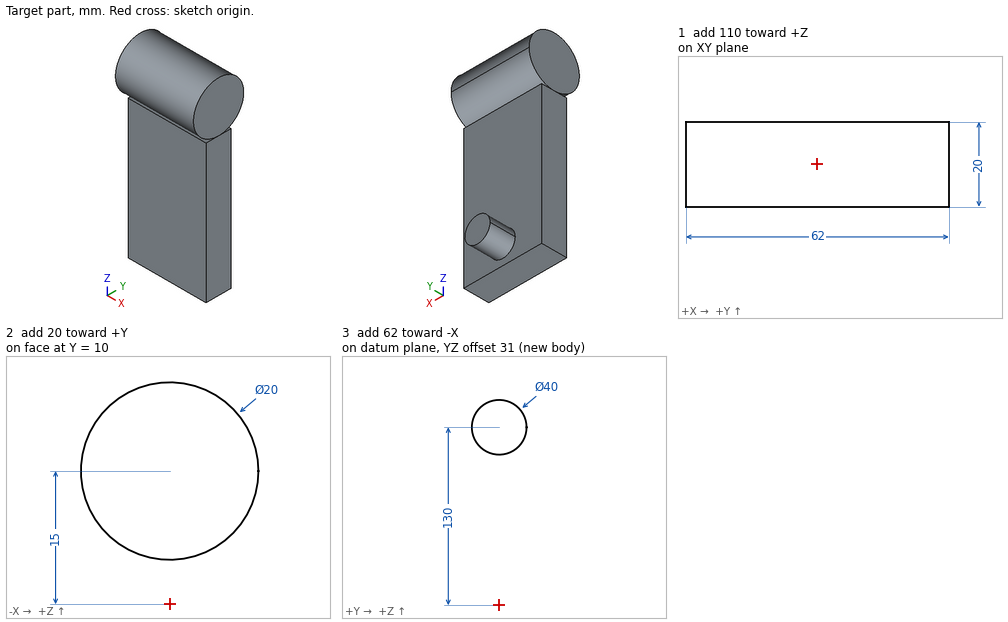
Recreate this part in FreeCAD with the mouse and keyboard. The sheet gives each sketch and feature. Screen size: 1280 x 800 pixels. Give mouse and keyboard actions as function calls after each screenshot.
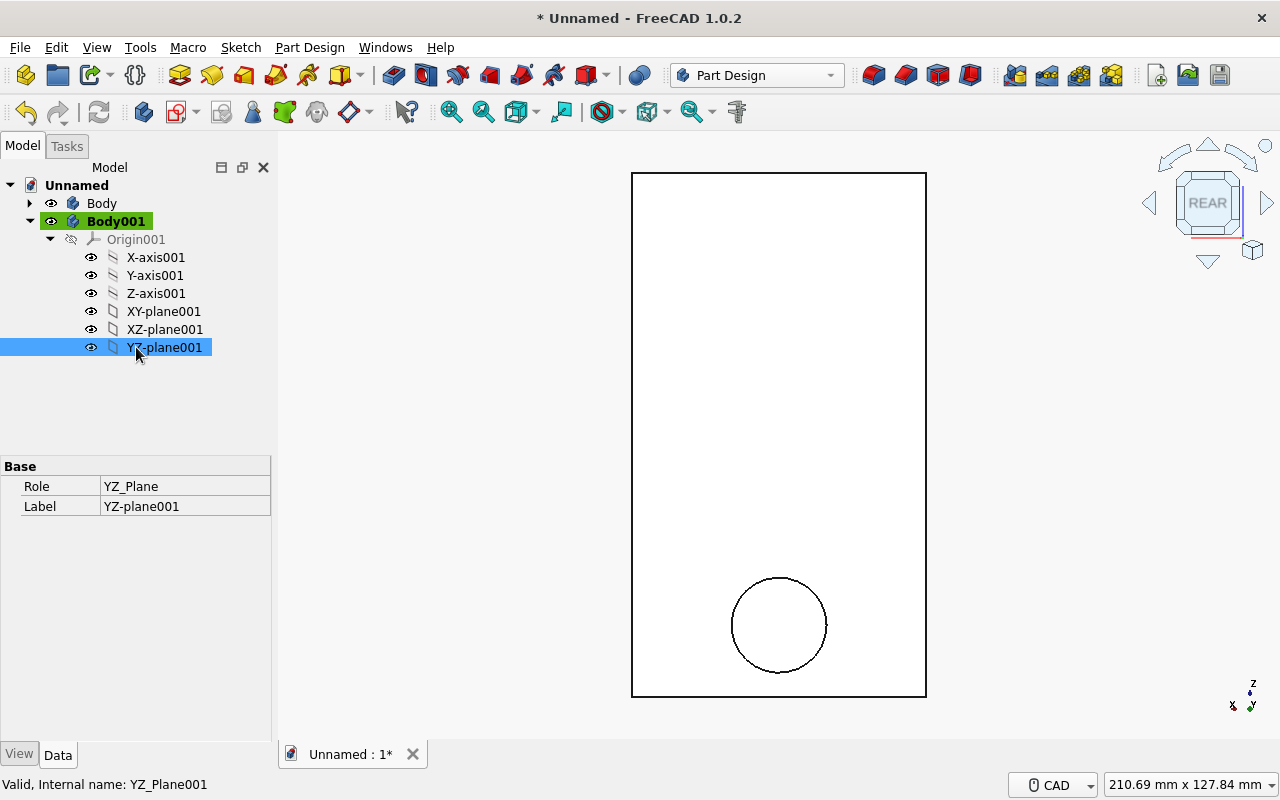
click(350, 112)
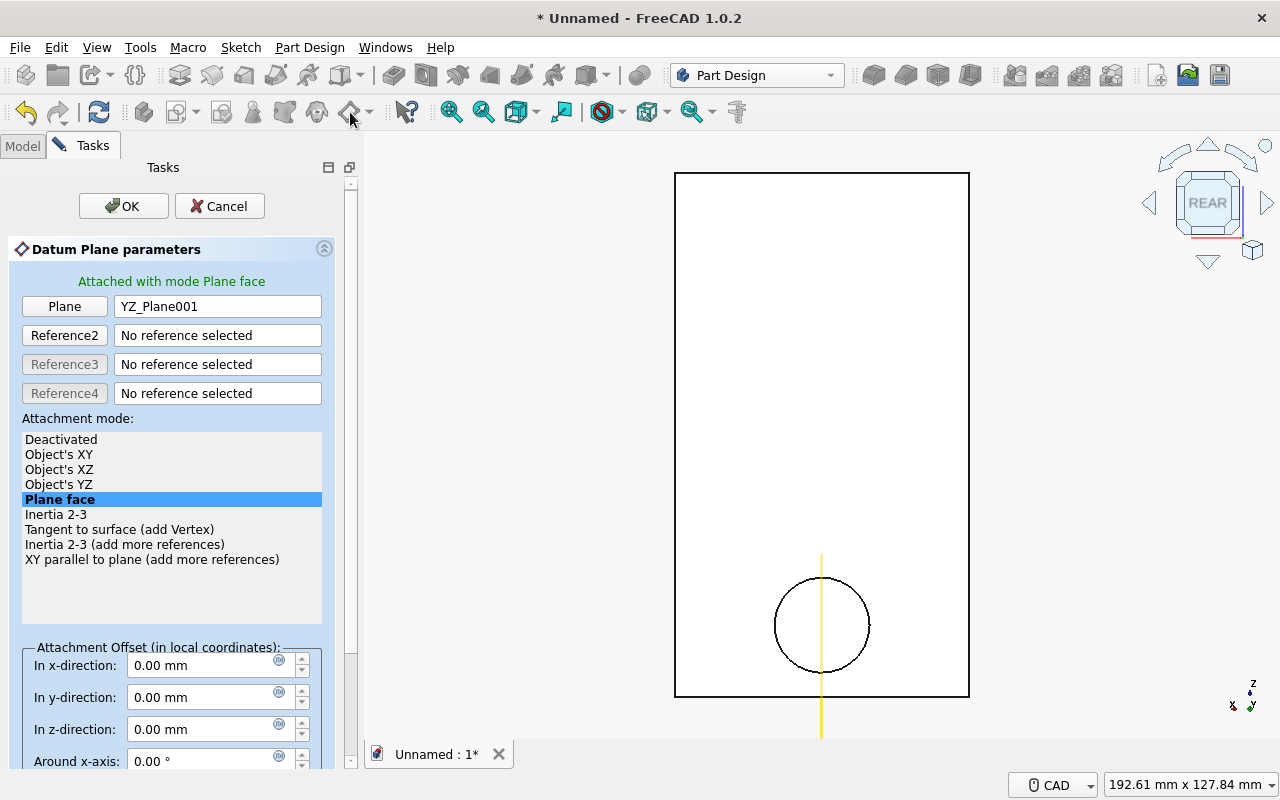
triple_click(210, 729)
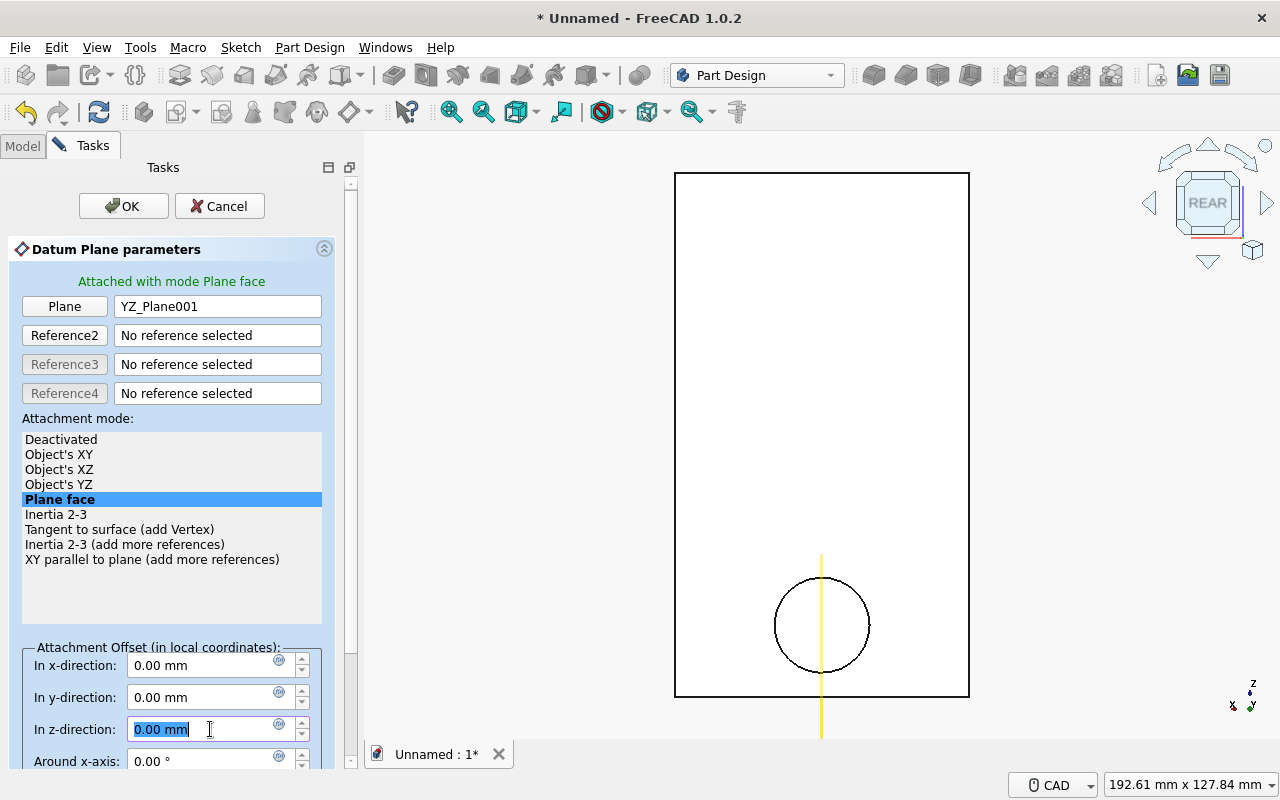
text(31)
key(Tab)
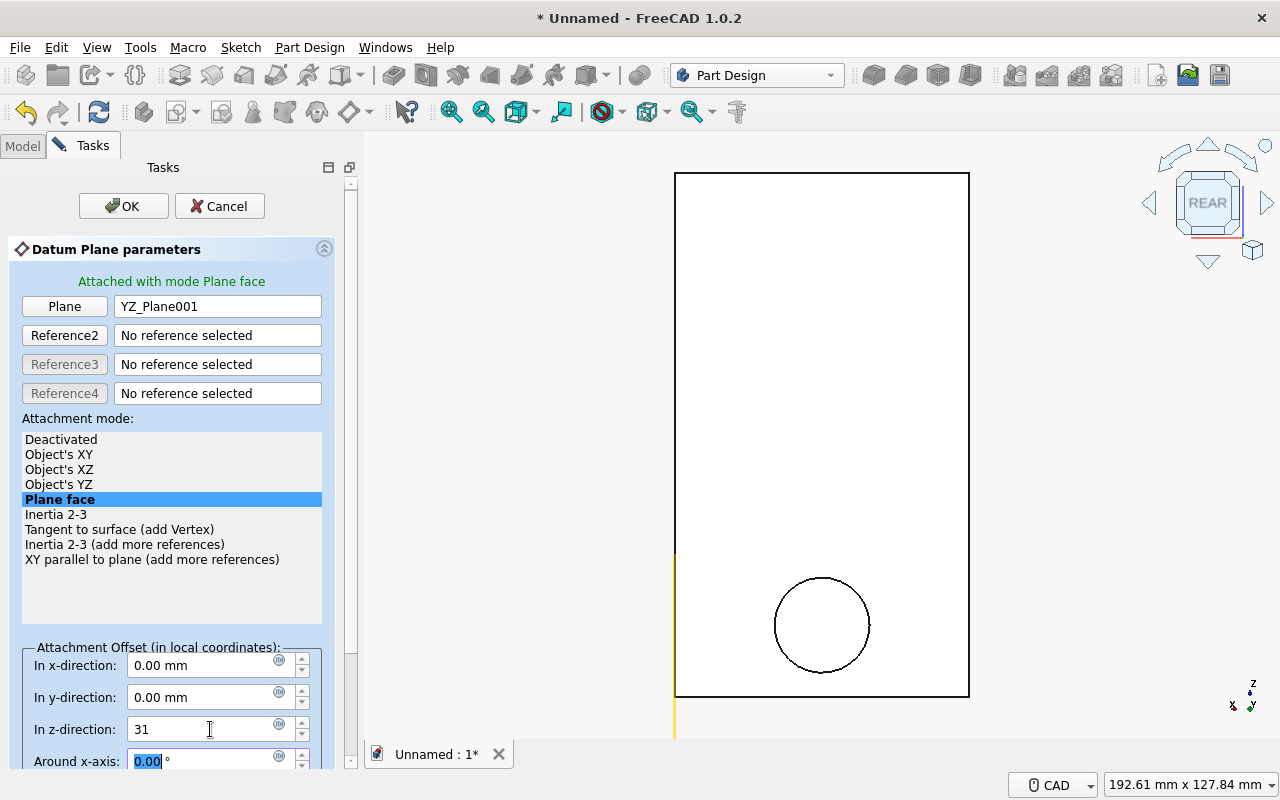
click(124, 206)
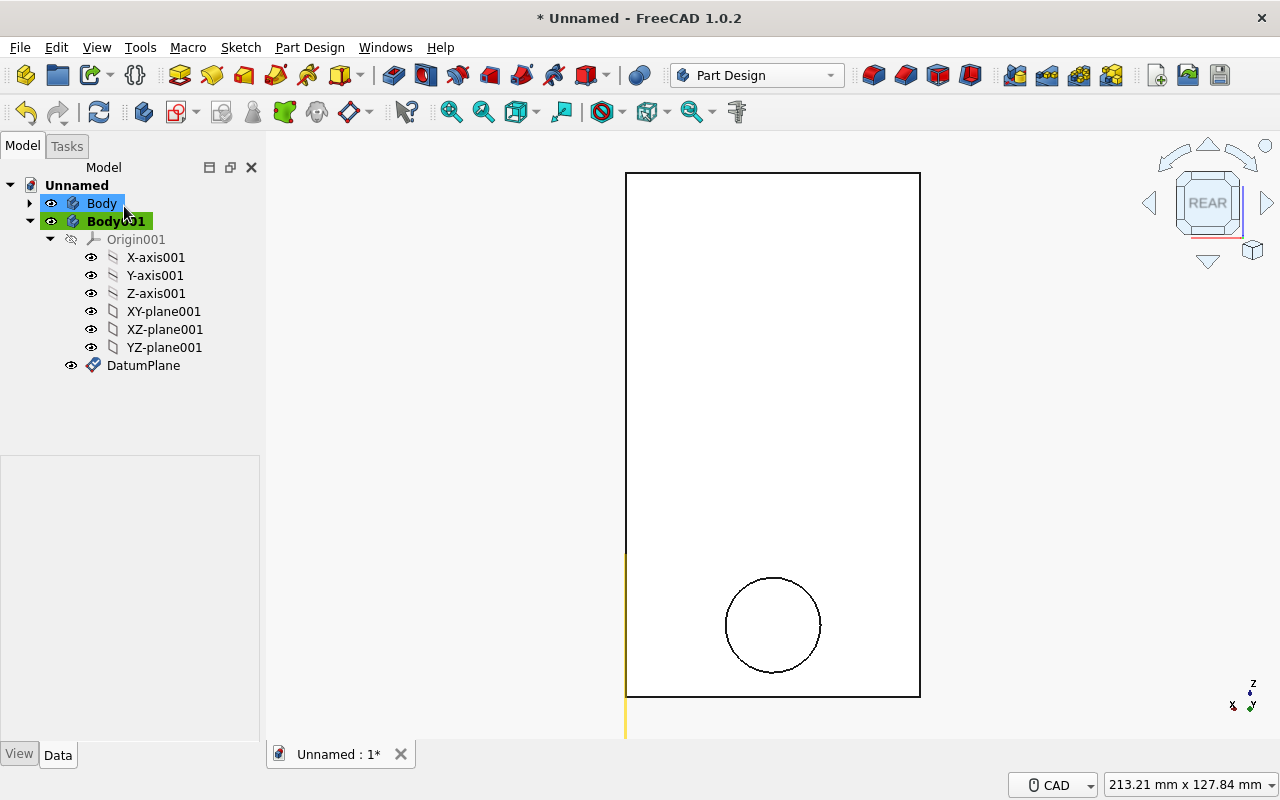
click(116, 365)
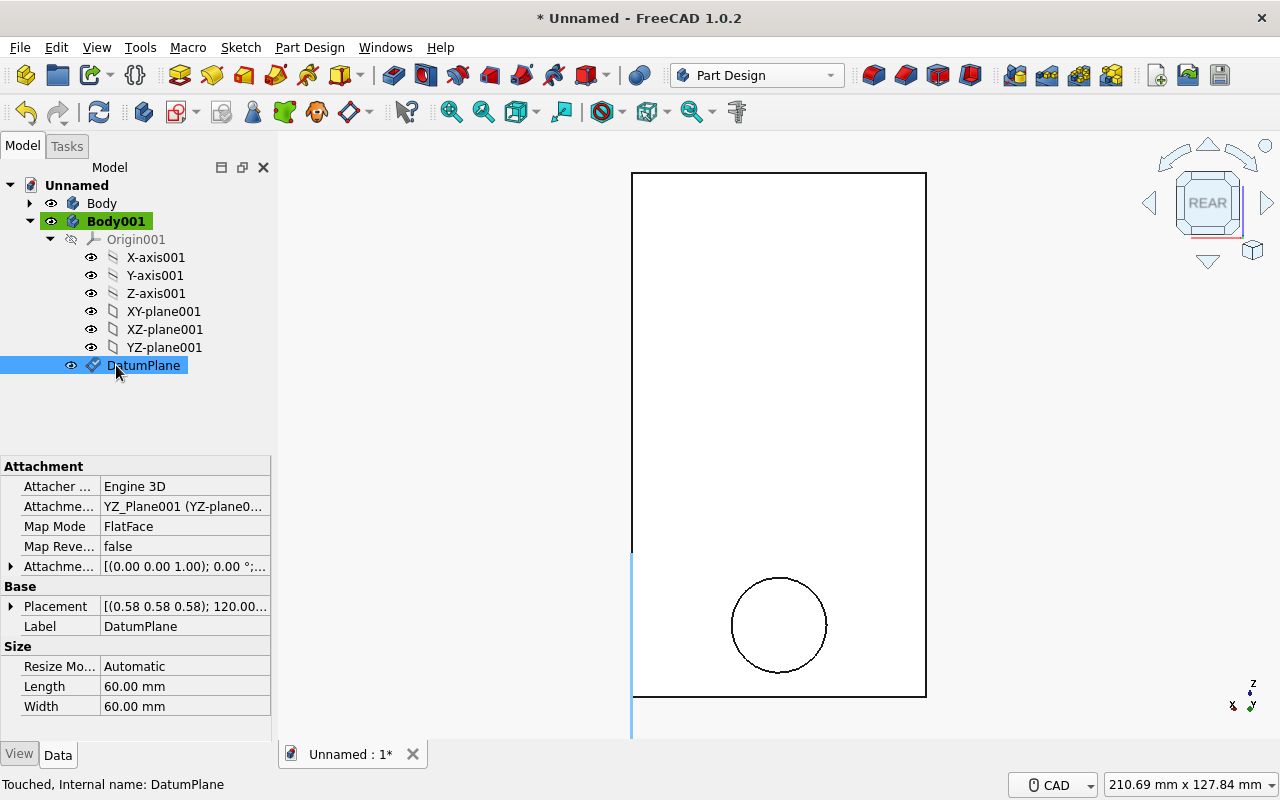
click(176, 112)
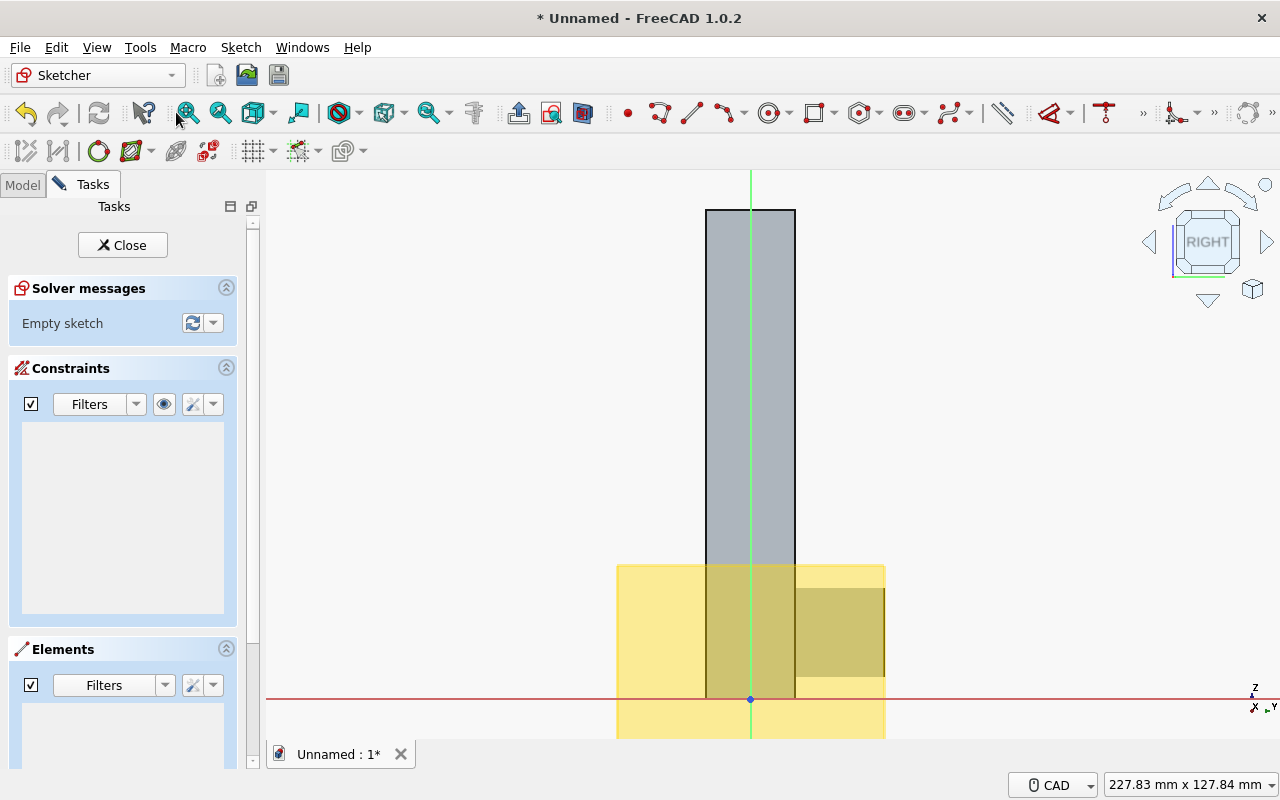
scroll(704, 454, down, 5)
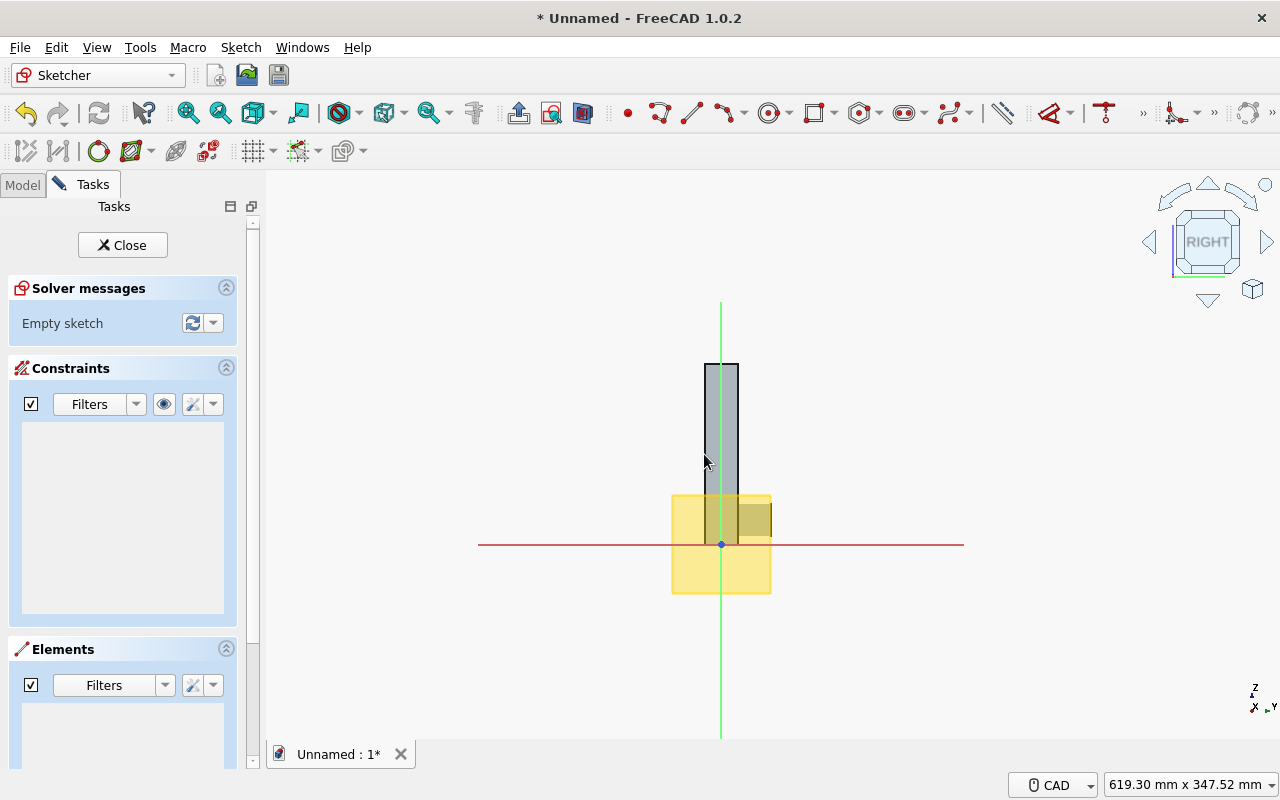
scroll(725, 307, up, 9)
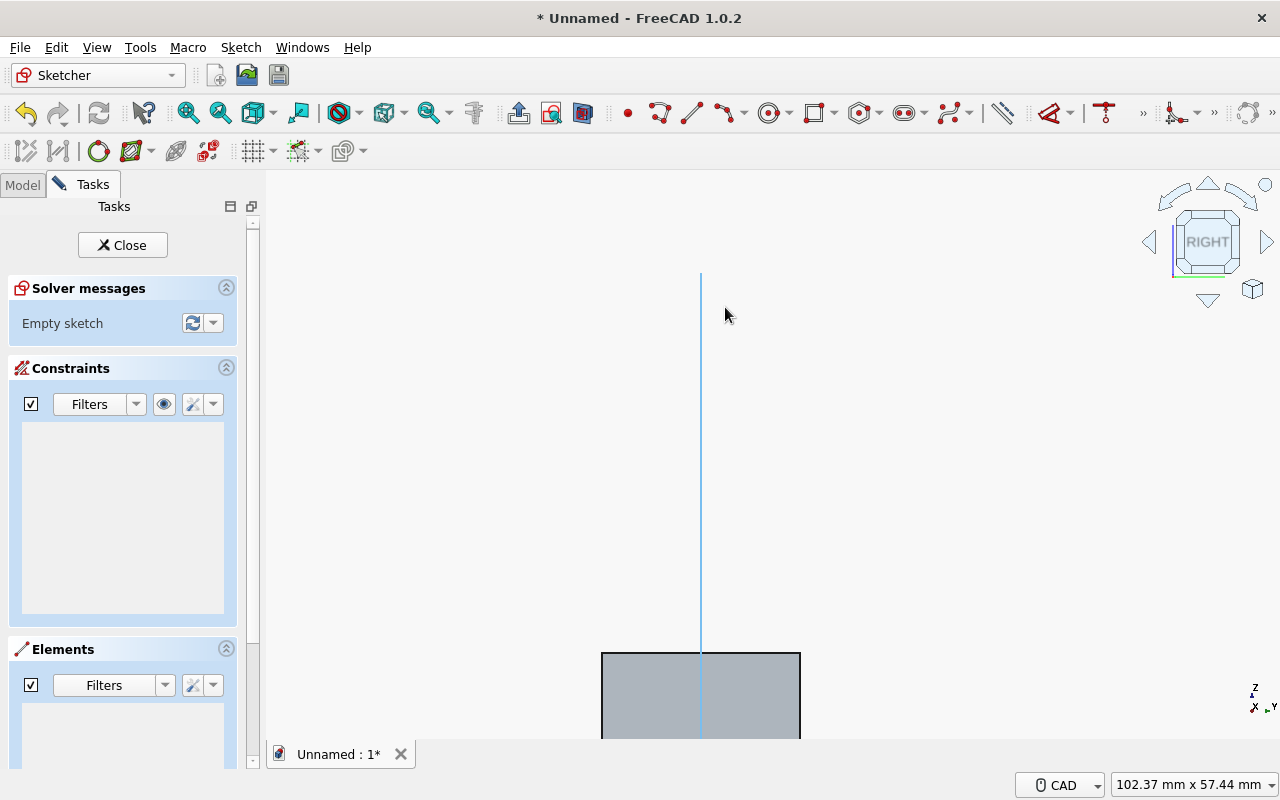
click(770, 114)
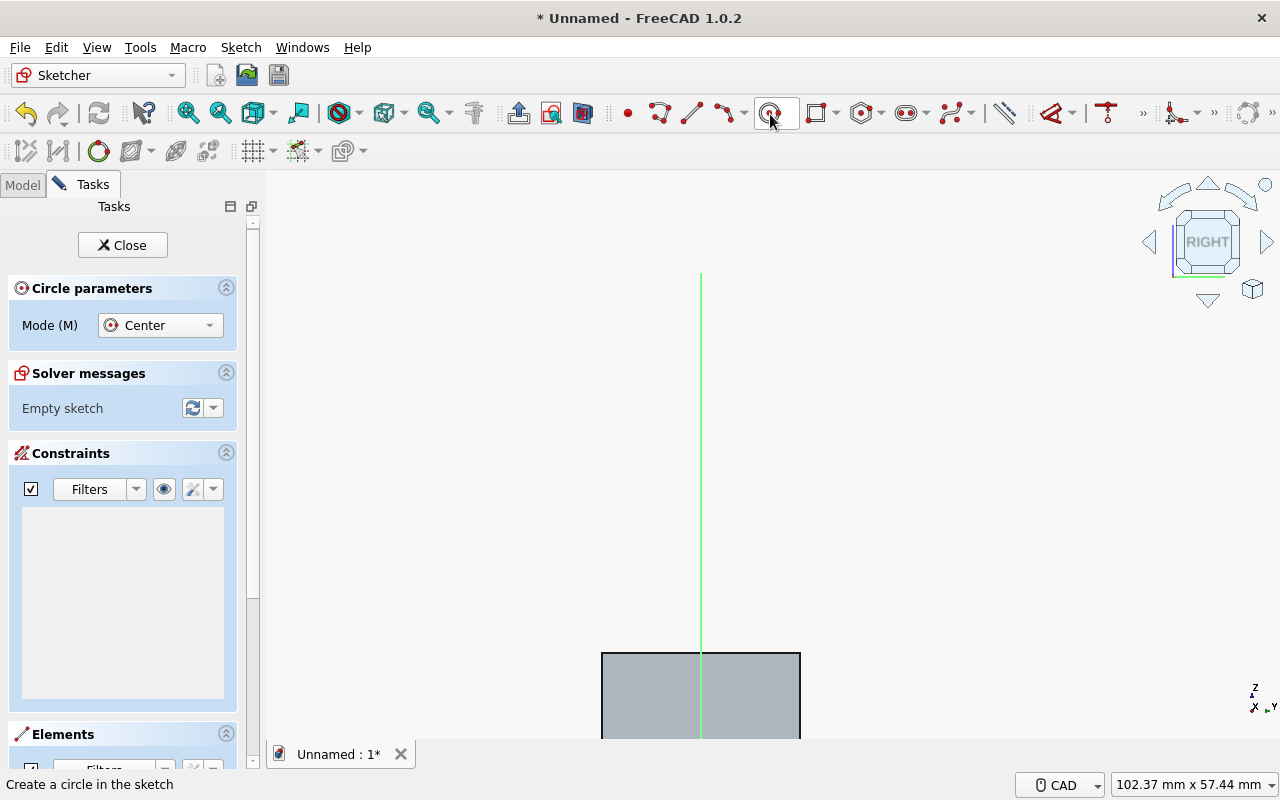
click(701, 455)
move(841, 315)